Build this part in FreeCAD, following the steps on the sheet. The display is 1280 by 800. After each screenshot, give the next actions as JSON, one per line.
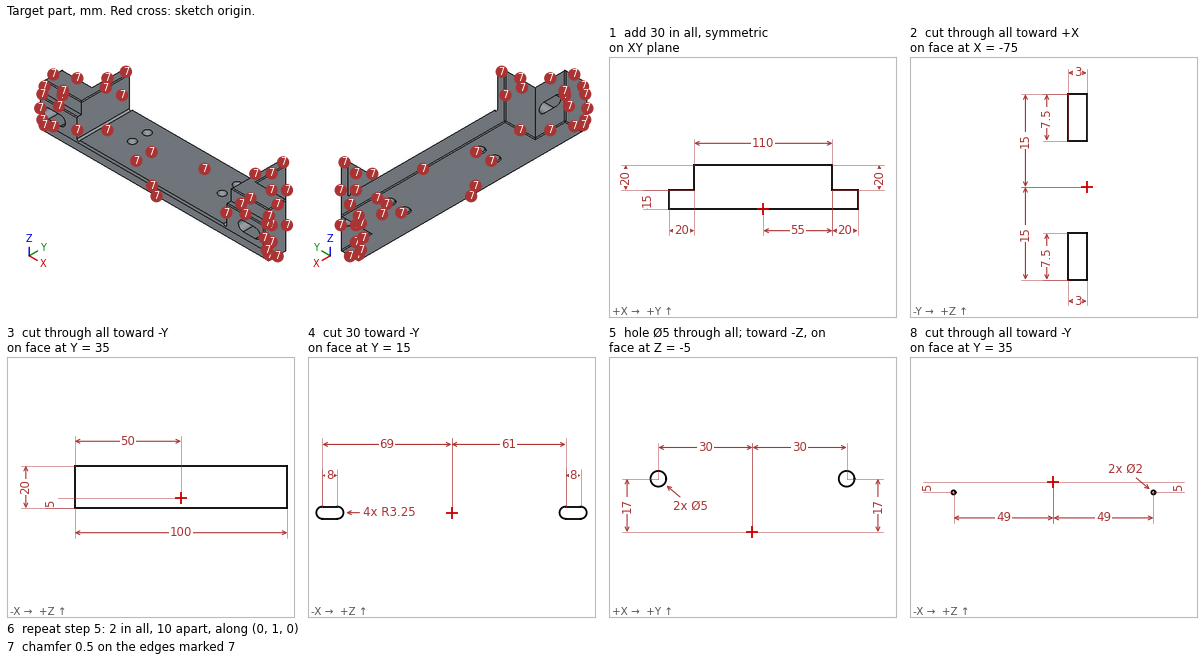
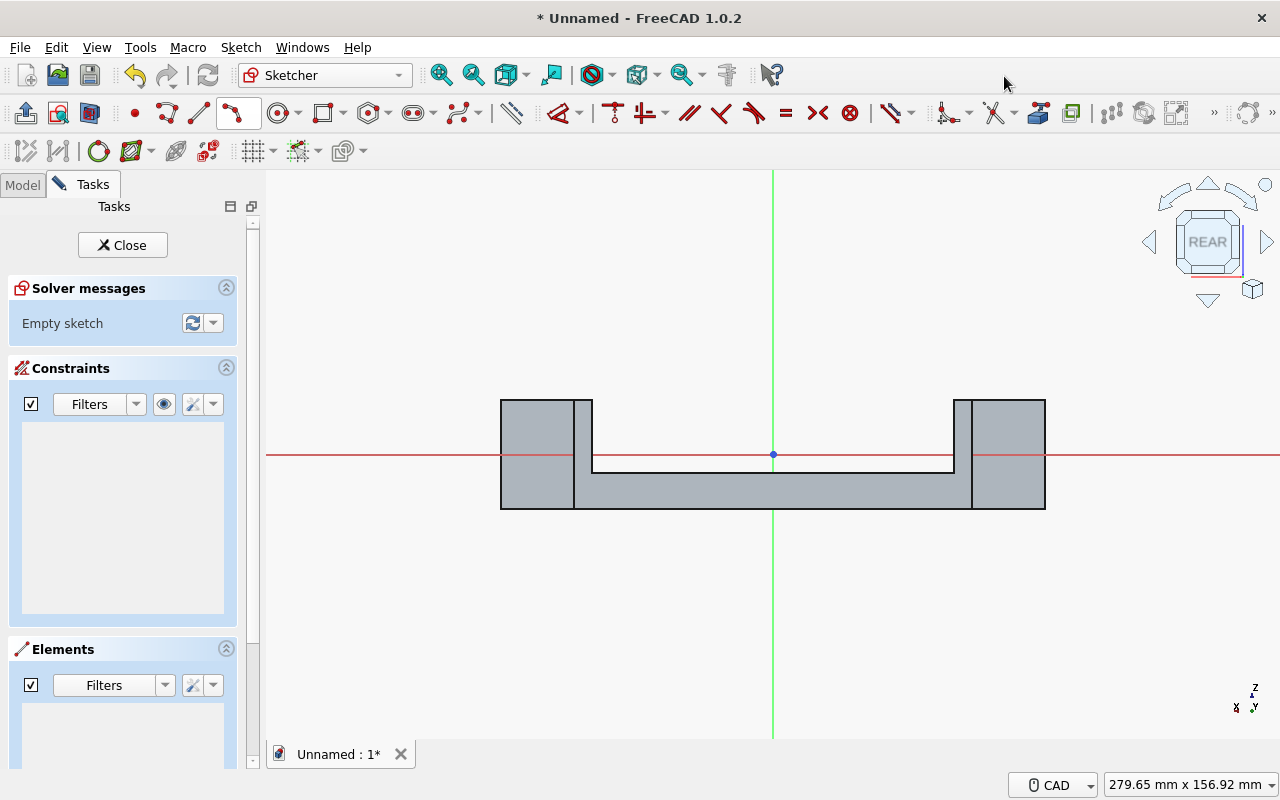
{"action": "key", "text": "q s"}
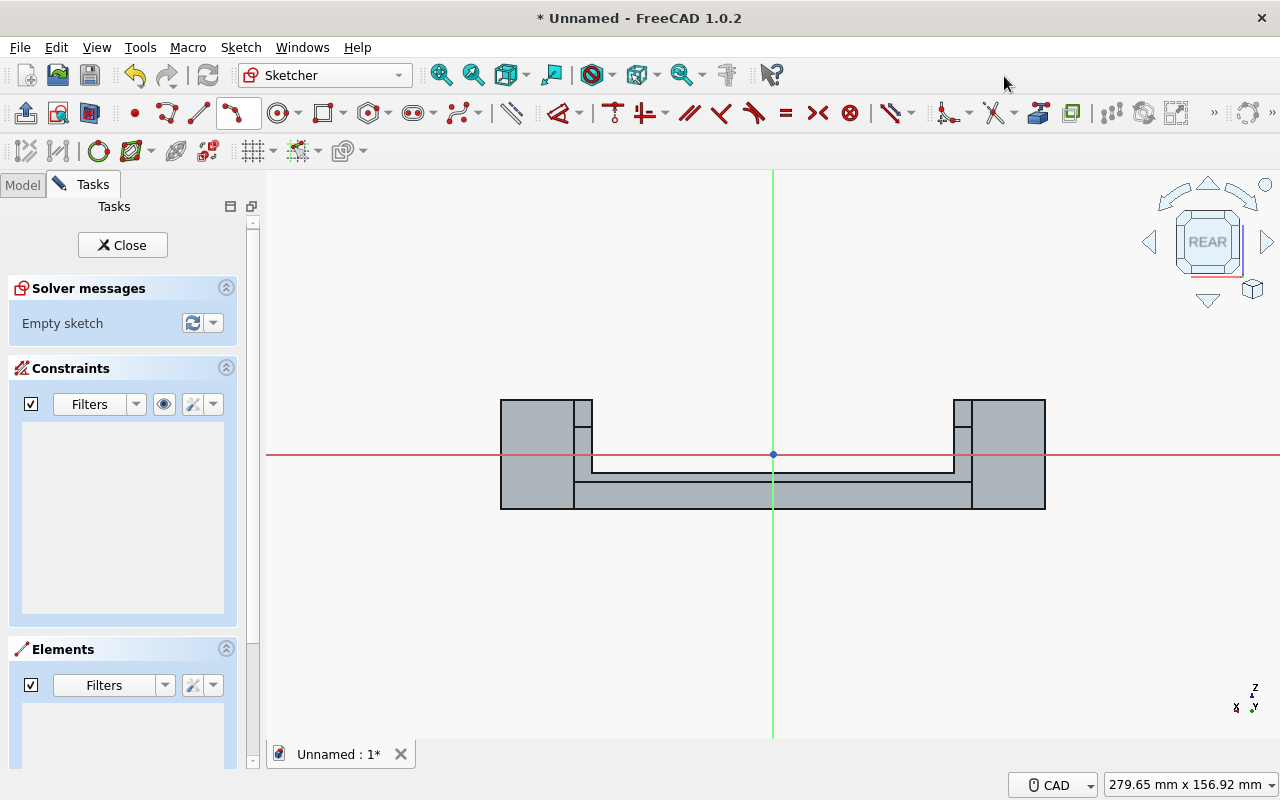
{"action": "key", "text": "g s"}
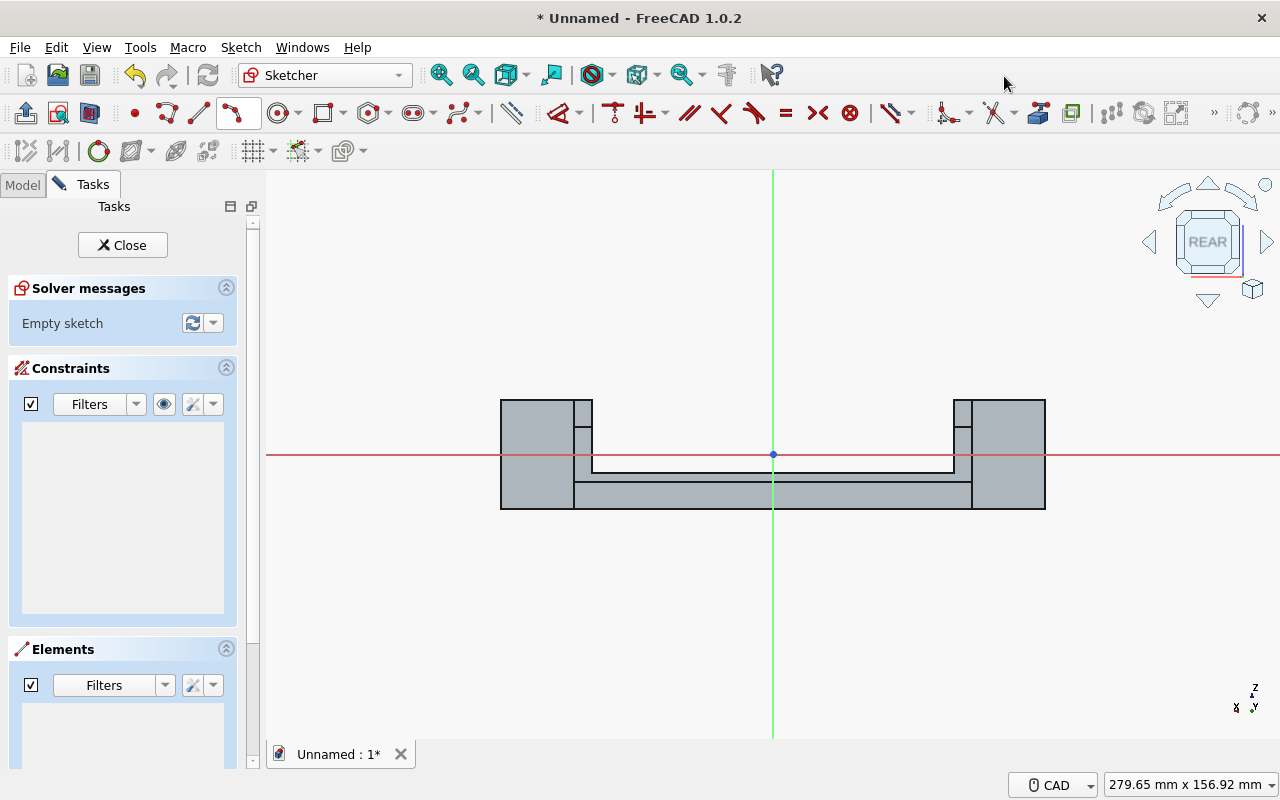
{"action": "scroll", "coordinate": [523, 455], "scroll_direction": "up", "scroll_amount": 4}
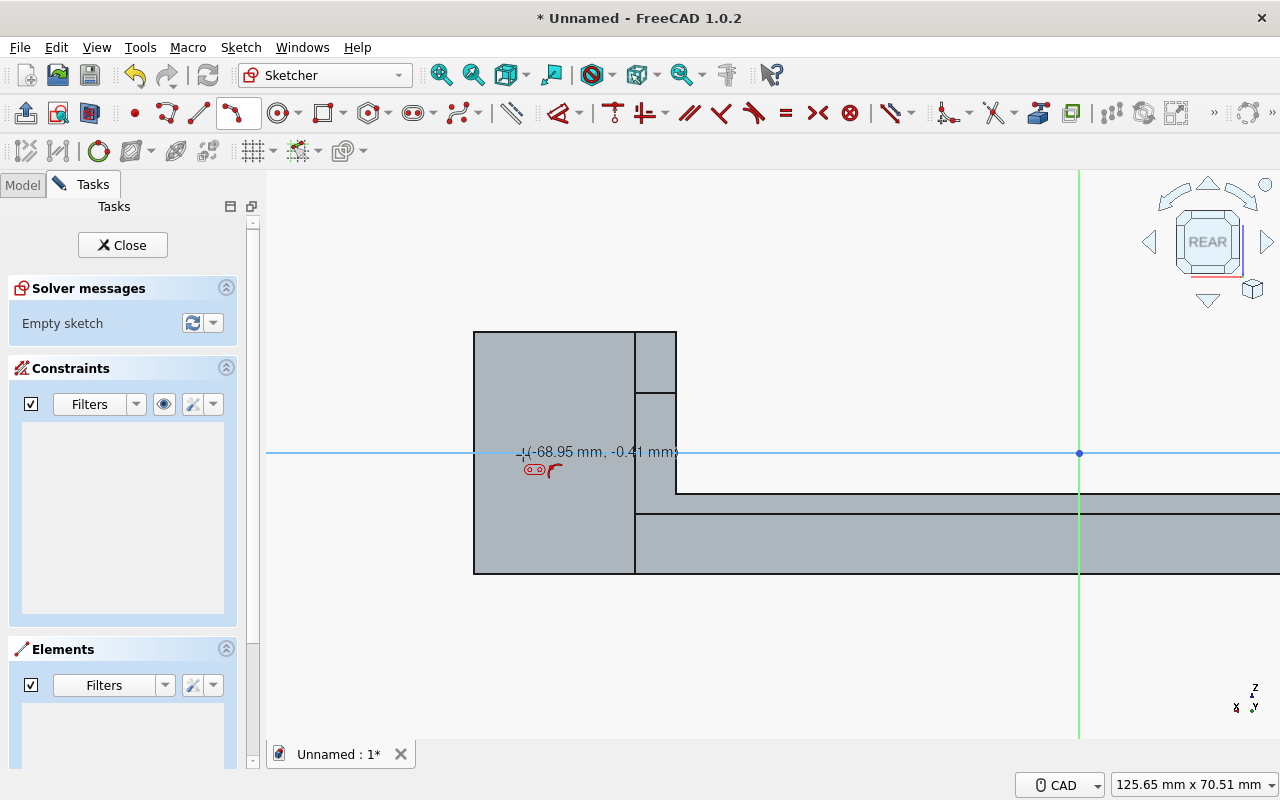
{"action": "left_click", "coordinate": [522, 453]}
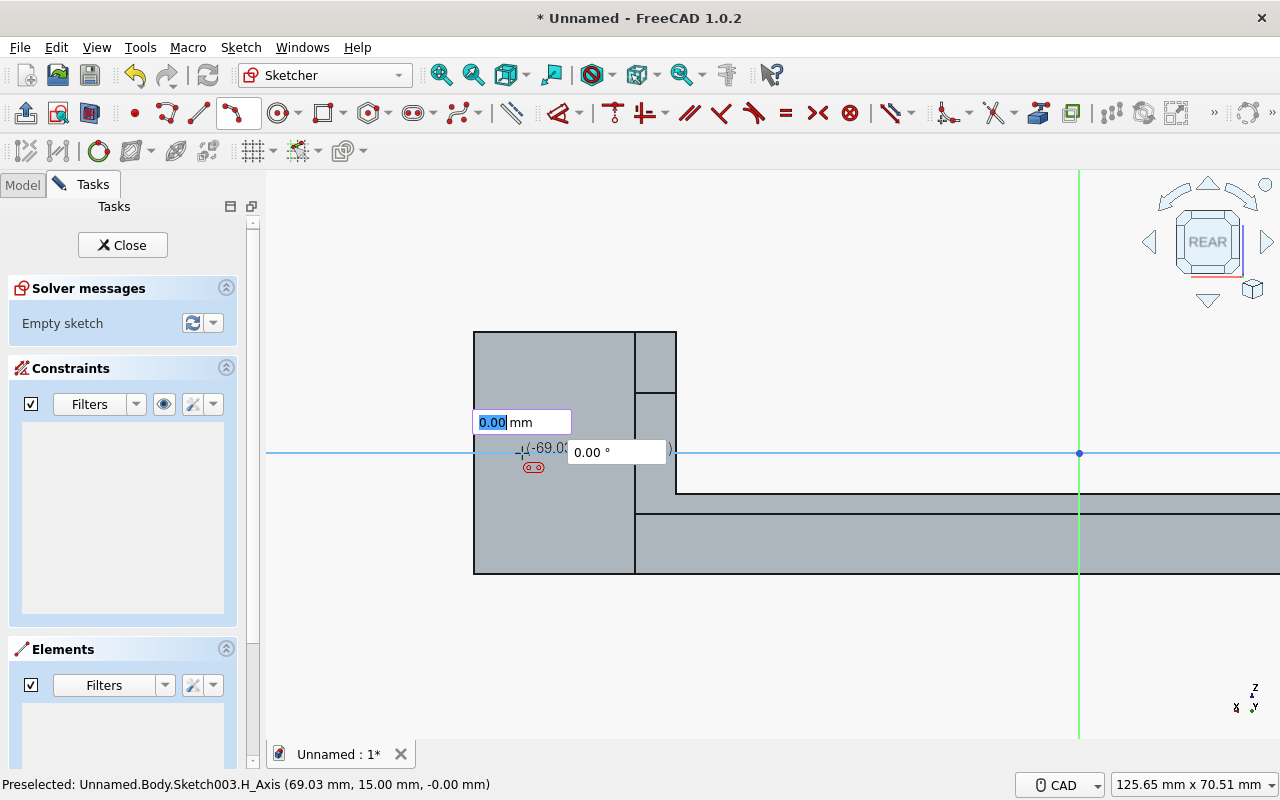
{"action": "left_click", "coordinate": [587, 444]}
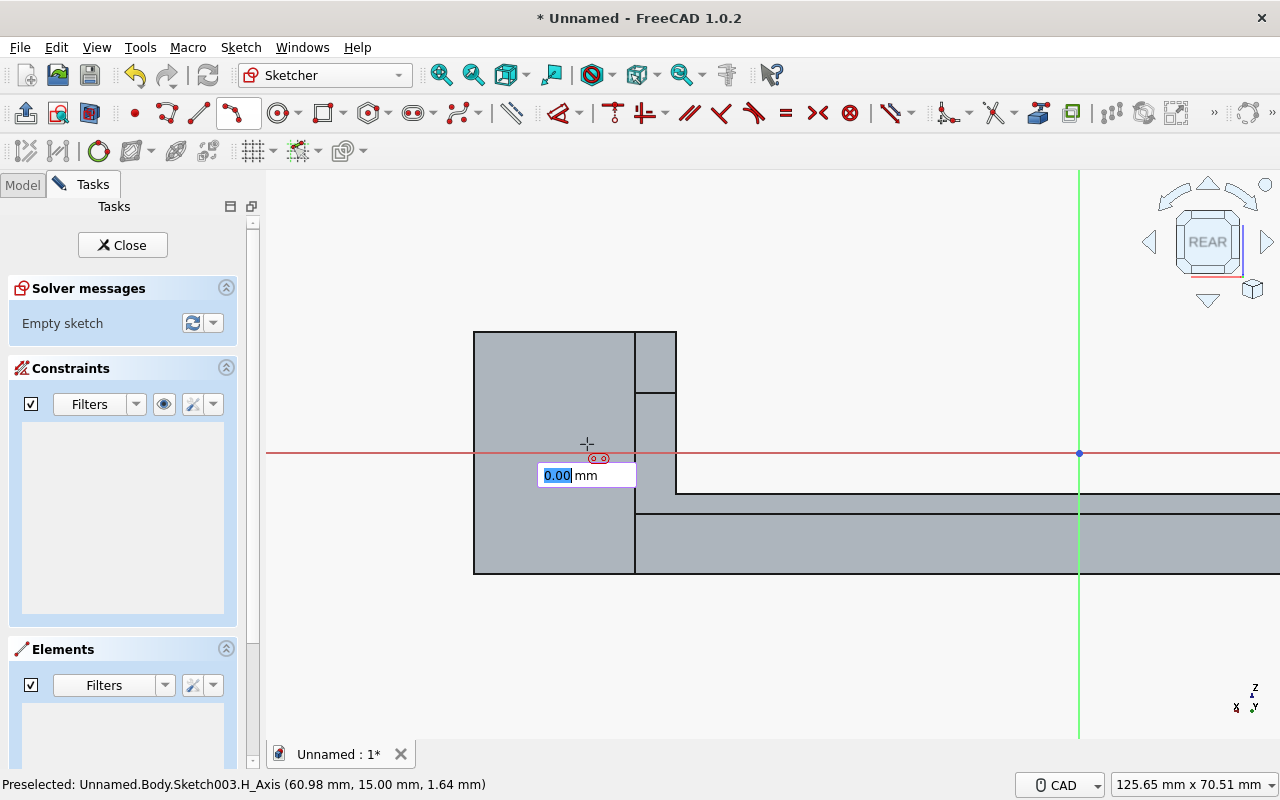
{"action": "left_click", "coordinate": [555, 479]}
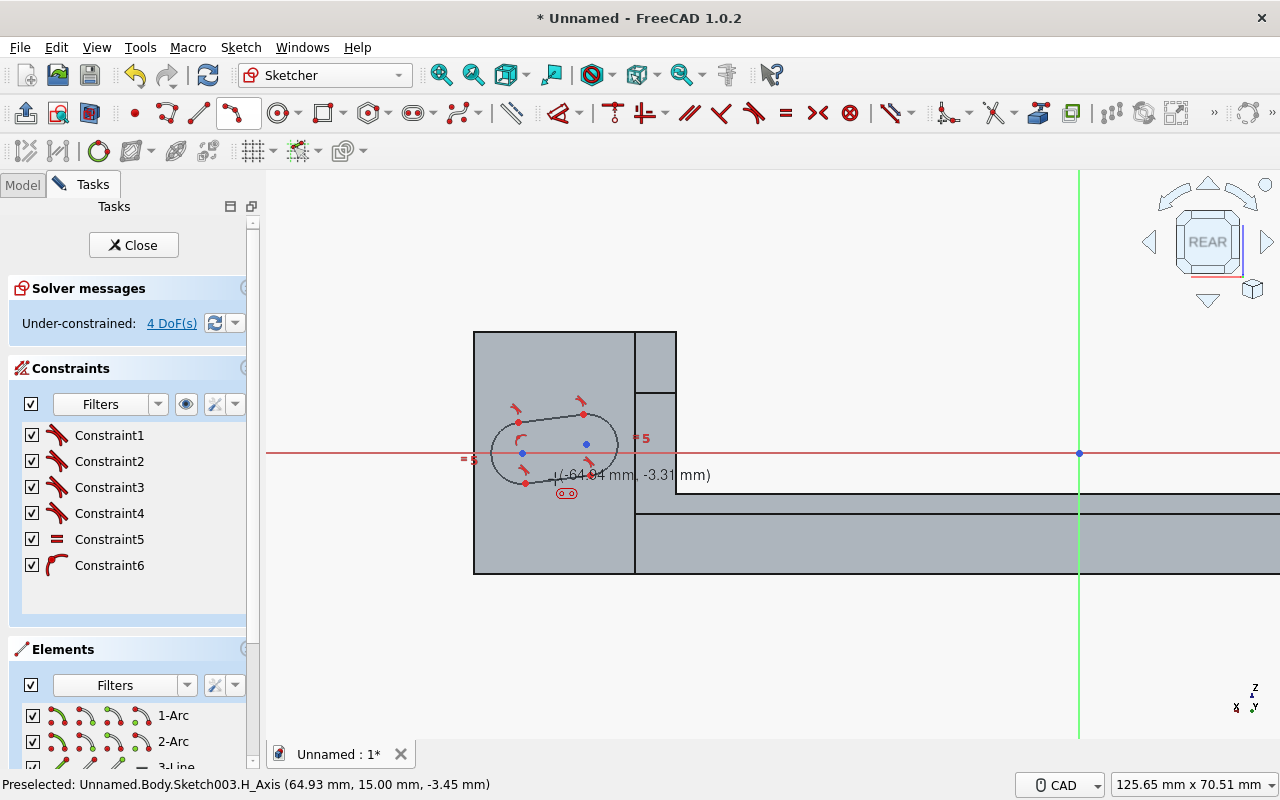
{"action": "scroll", "coordinate": [294, 456], "scroll_direction": "down", "scroll_amount": 3}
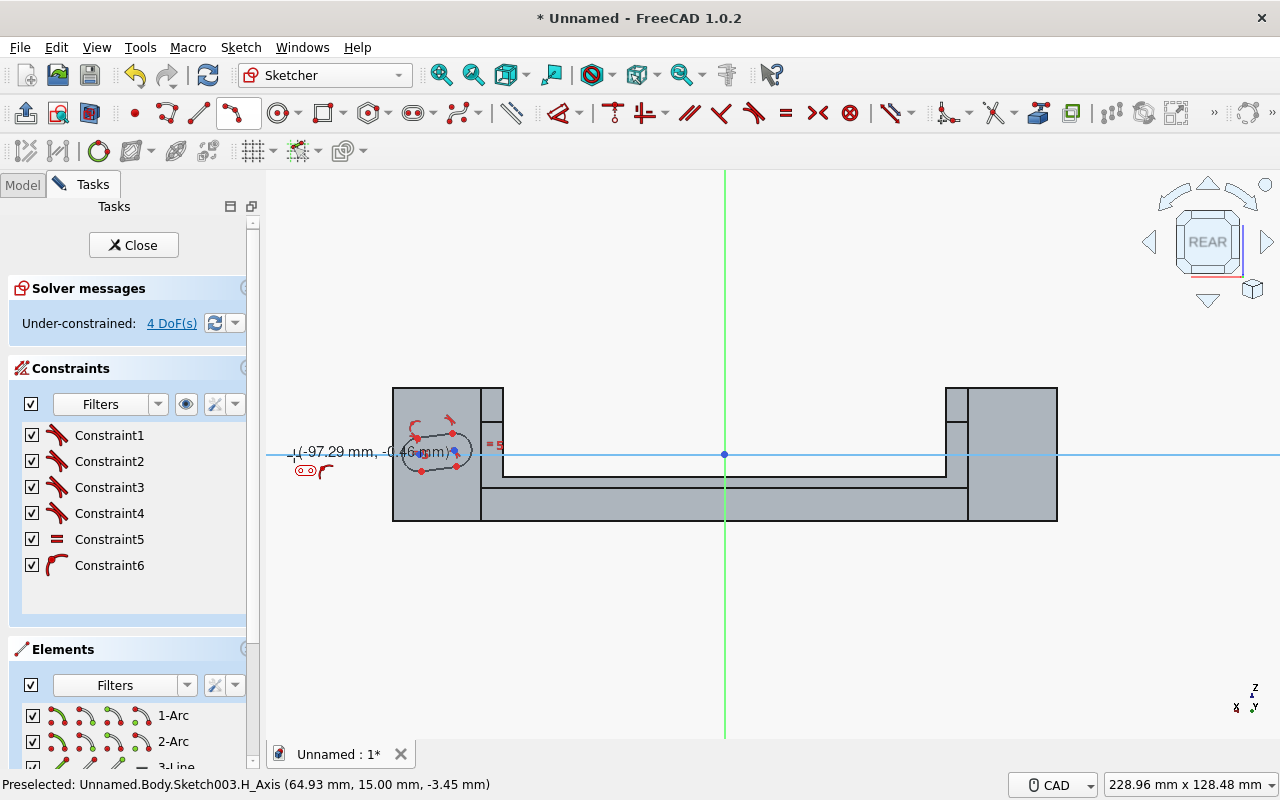
{"action": "scroll", "coordinate": [995, 455], "scroll_direction": "up", "scroll_amount": 3}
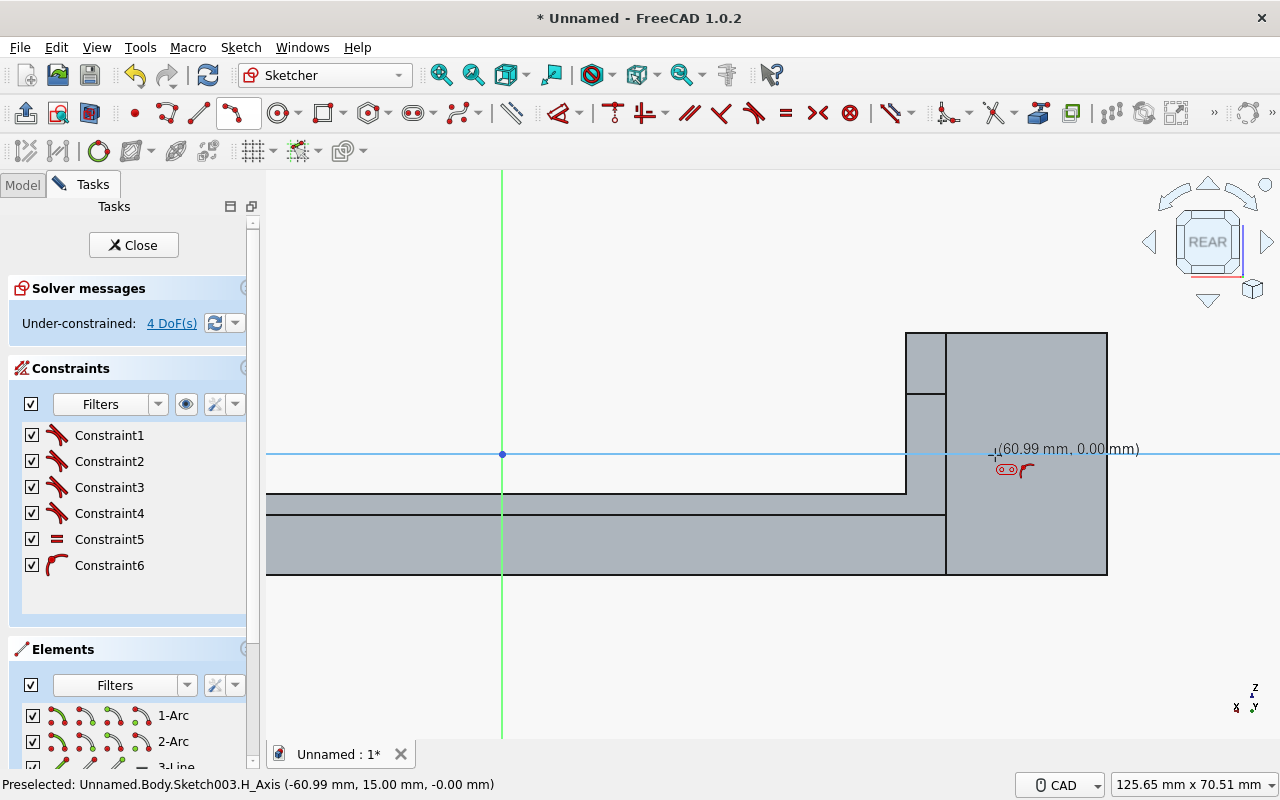
{"action": "left_click", "coordinate": [994, 454]}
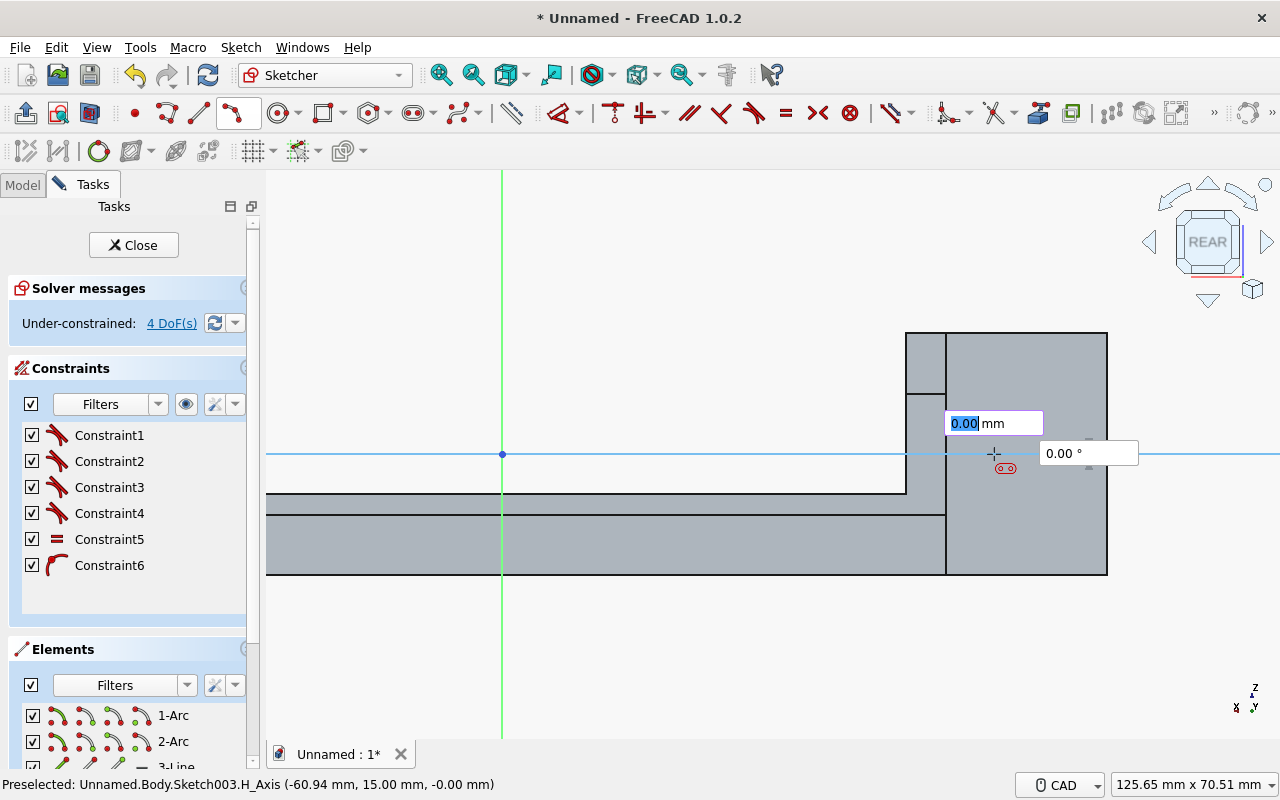
{"action": "left_click", "coordinate": [1059, 445]}